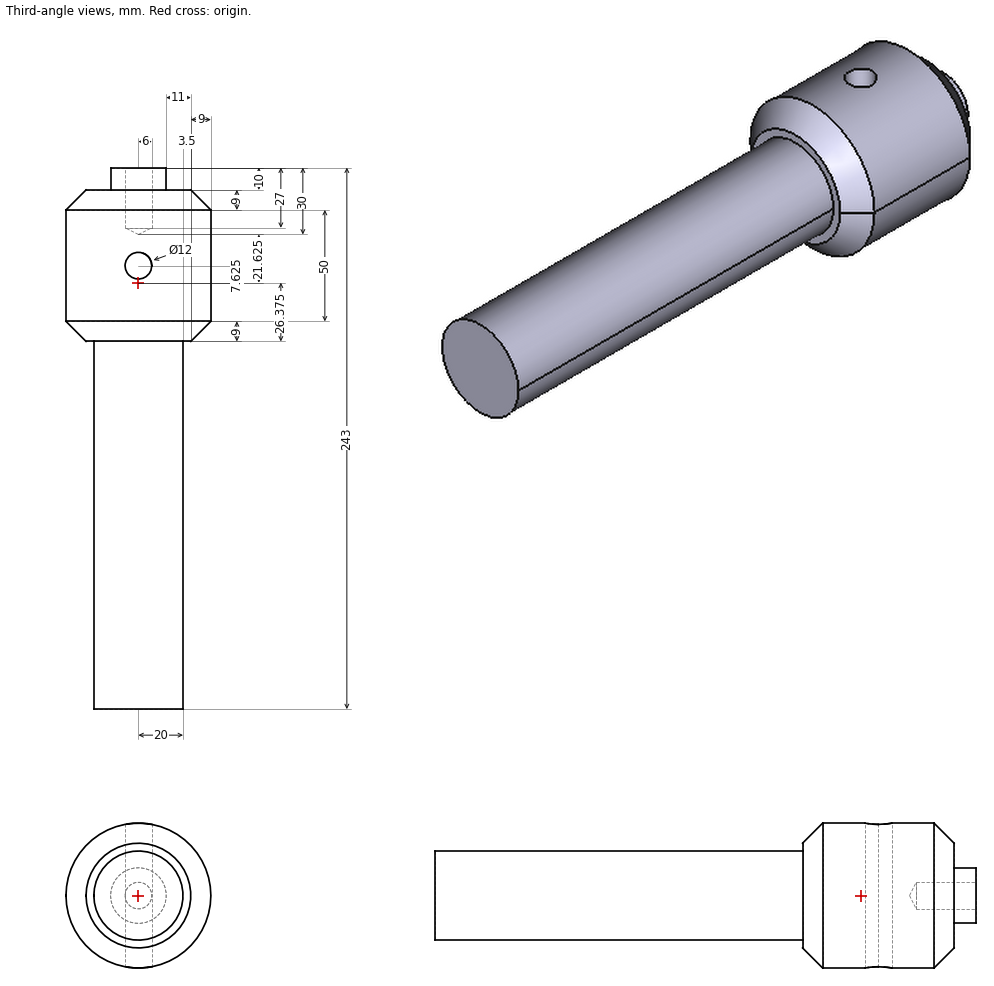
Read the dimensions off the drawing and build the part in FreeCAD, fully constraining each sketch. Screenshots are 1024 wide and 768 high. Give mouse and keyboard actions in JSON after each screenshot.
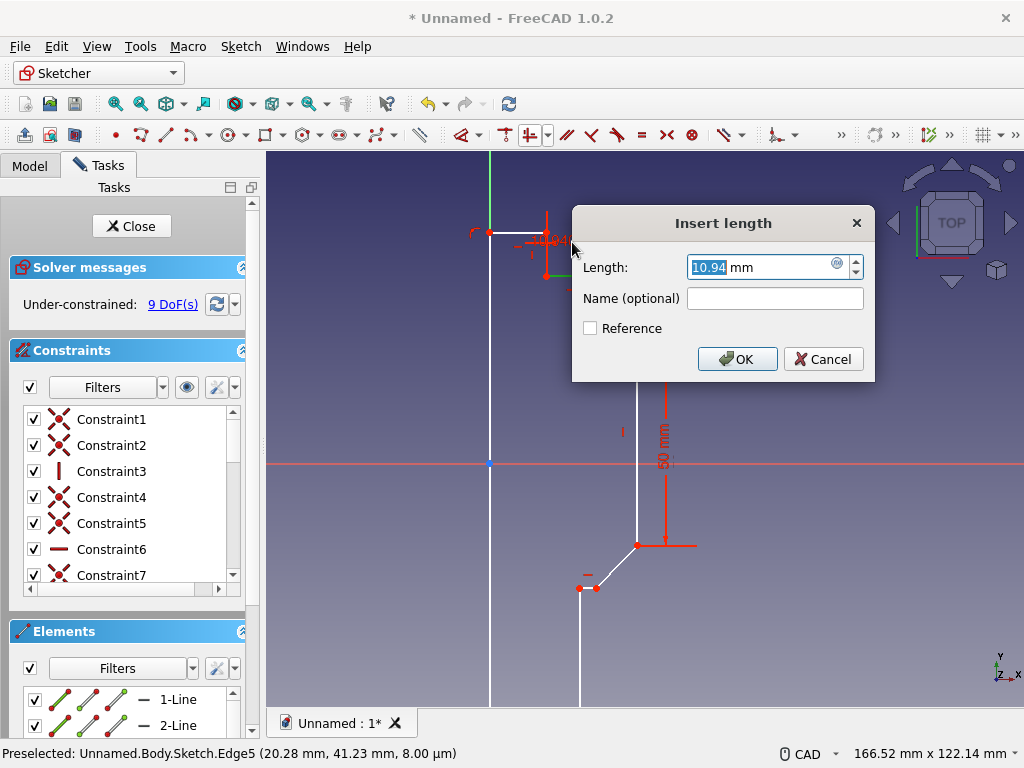
{"action": "type", "text": "11"}
{"action": "key", "text": "Return"}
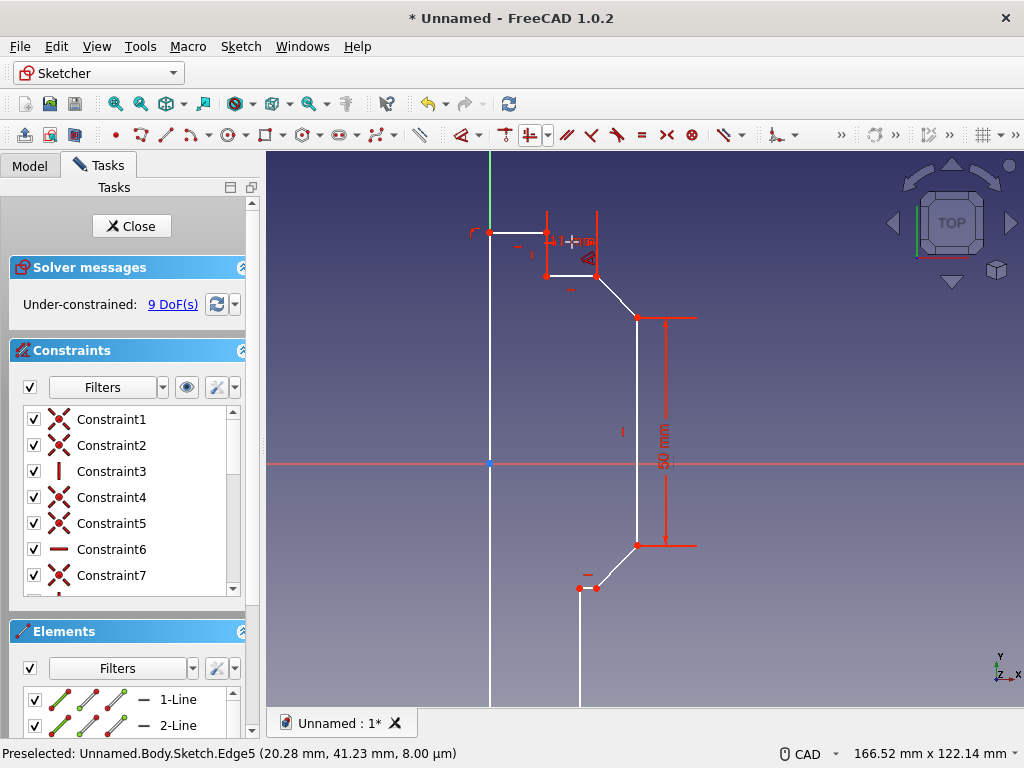
{"action": "left_click", "coordinate": [547, 263]}
{"action": "left_click", "coordinate": [513, 264]}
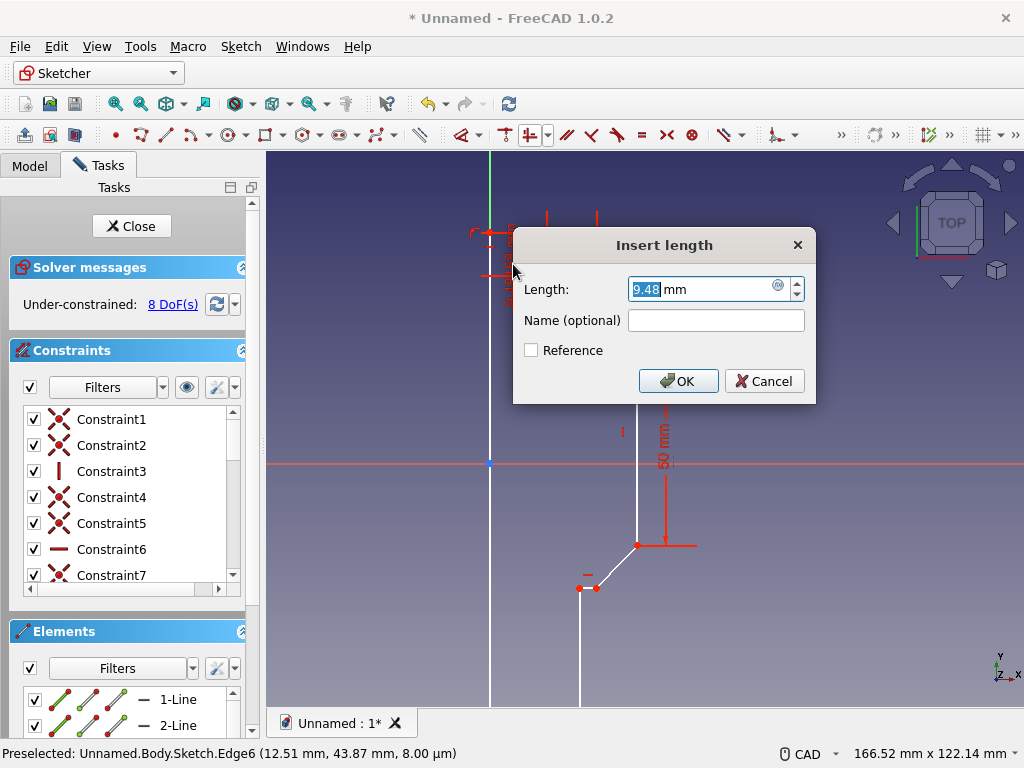
{"action": "type", "text": "10"}
{"action": "key", "text": "Return"}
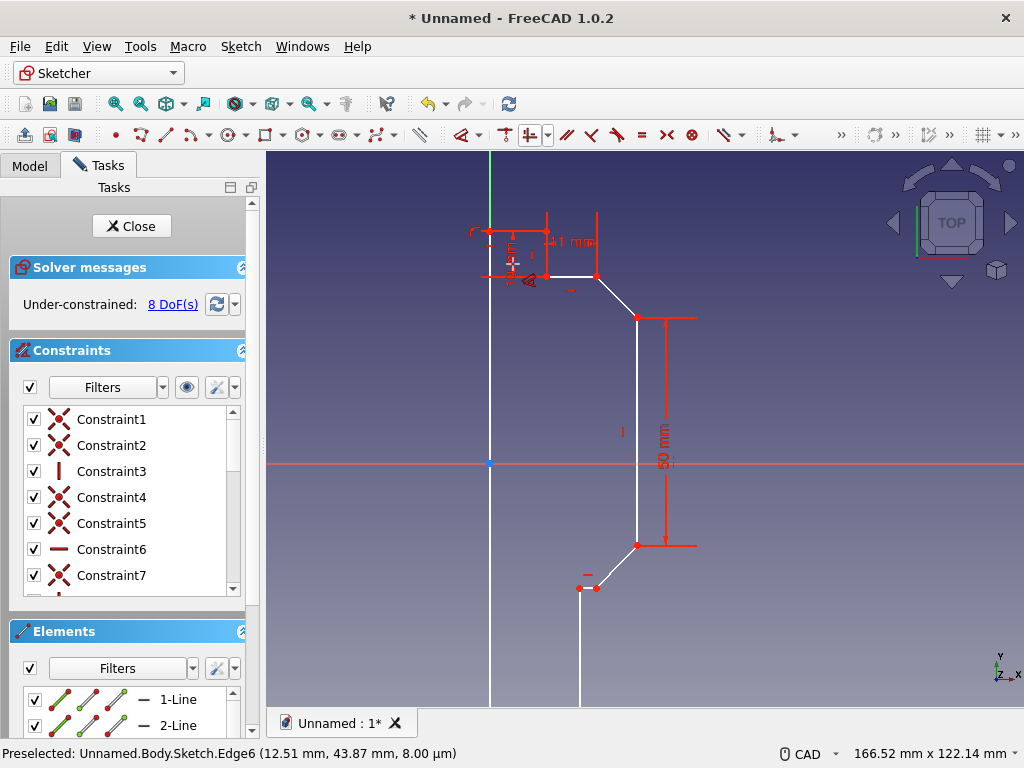
{"action": "scroll", "coordinate": [582, 277], "scroll_direction": "down", "scroll_amount": 6}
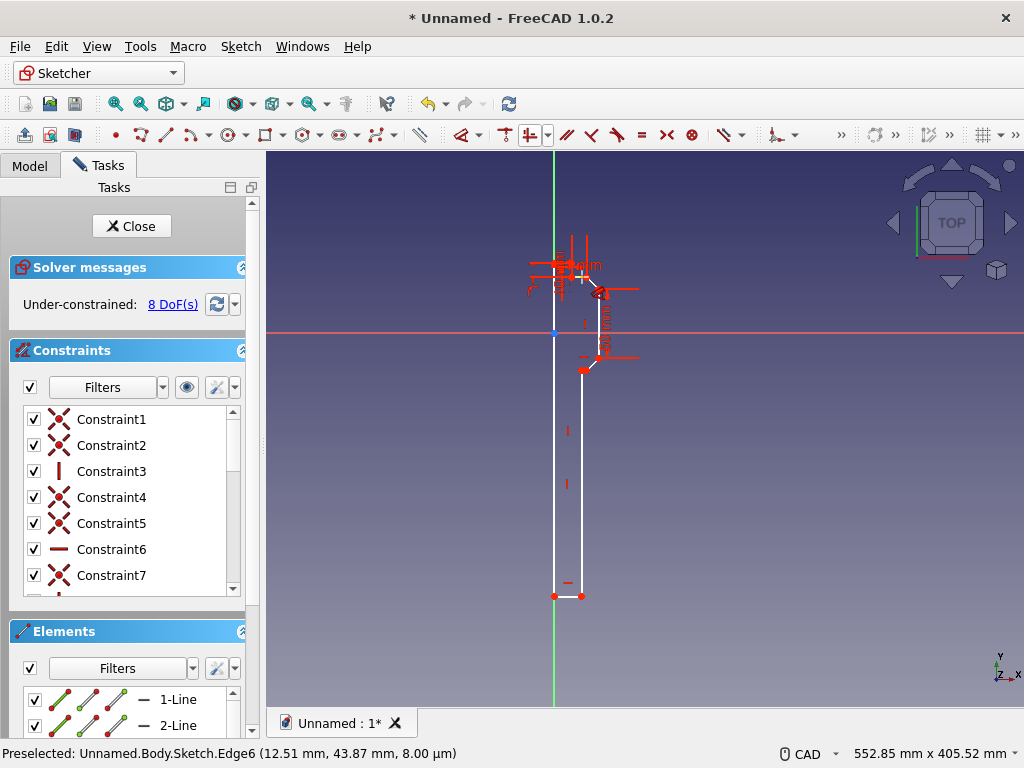
{"action": "scroll", "coordinate": [563, 597], "scroll_direction": "up", "scroll_amount": 3}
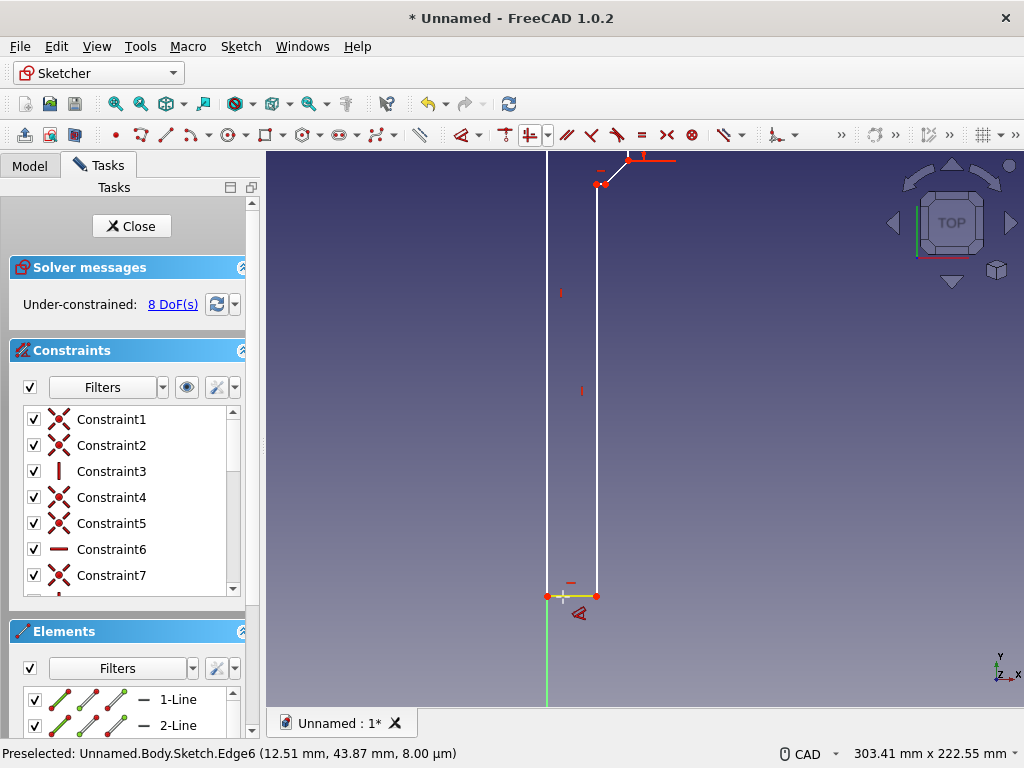
{"action": "left_click", "coordinate": [562, 596]}
{"action": "left_click", "coordinate": [572, 630]}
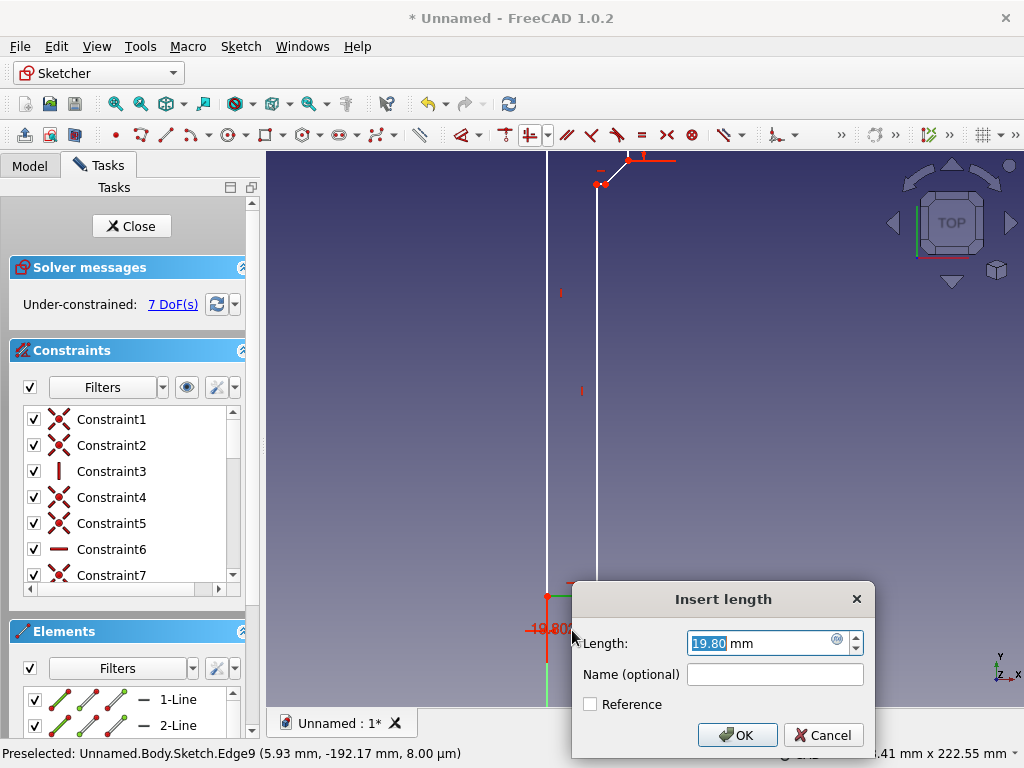
{"action": "type", "text": "20"}
{"action": "key", "text": "Return"}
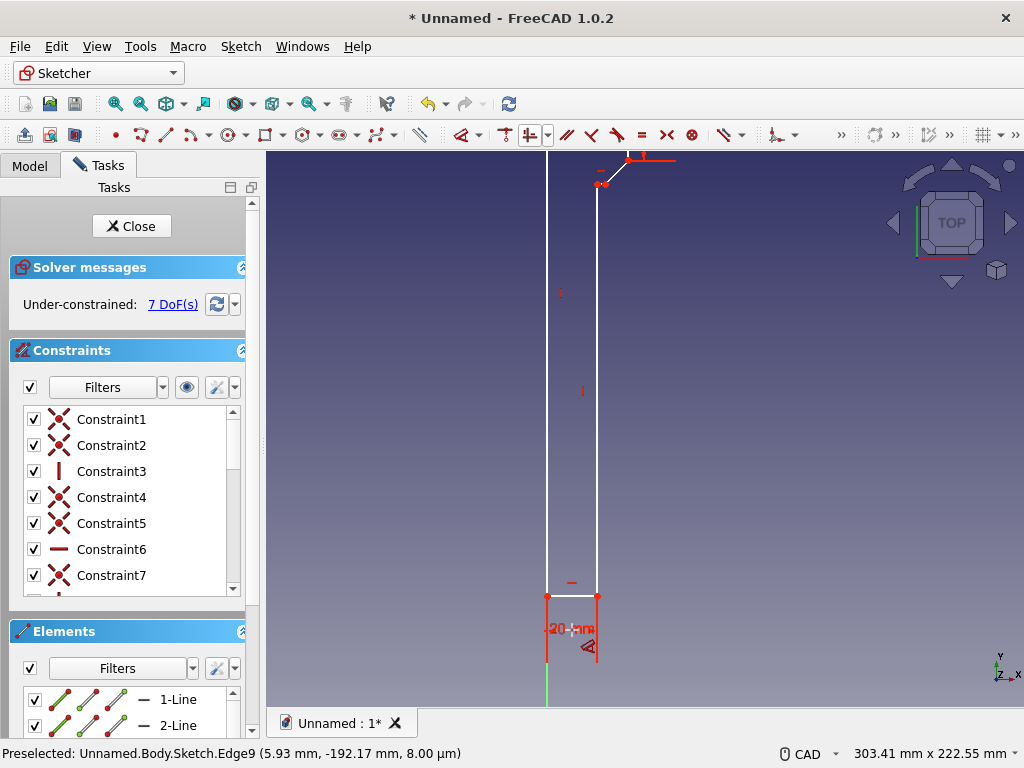
{"action": "scroll", "coordinate": [563, 597], "scroll_direction": "down", "scroll_amount": 3}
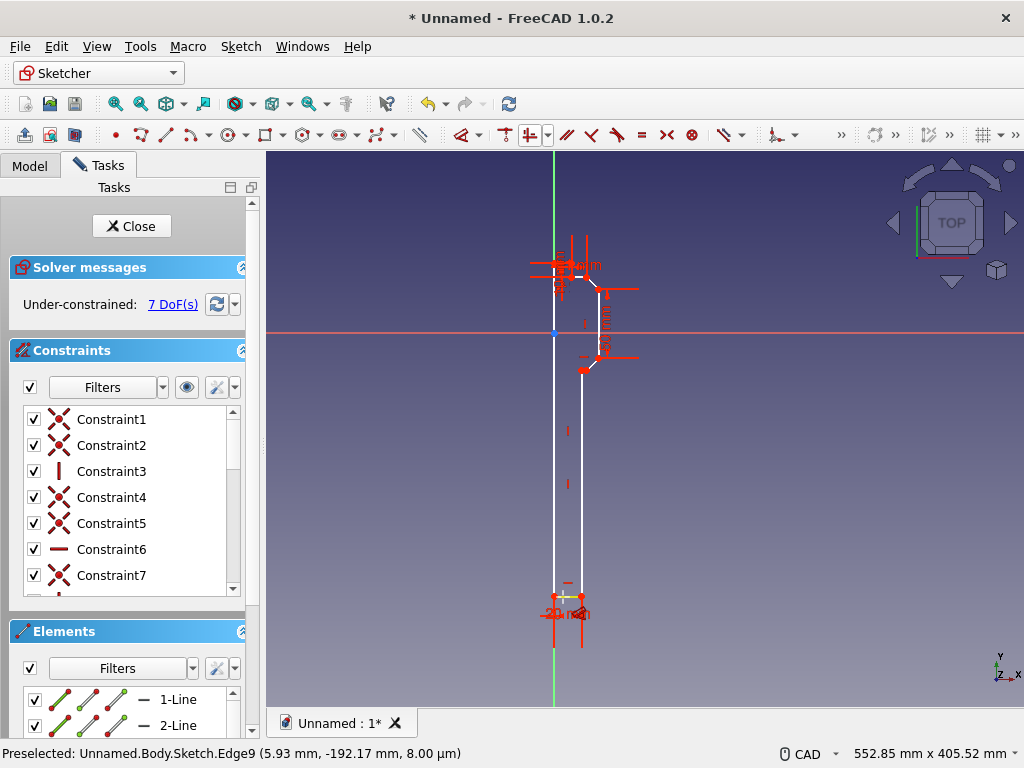
{"action": "scroll", "coordinate": [590, 367], "scroll_direction": "up", "scroll_amount": 6}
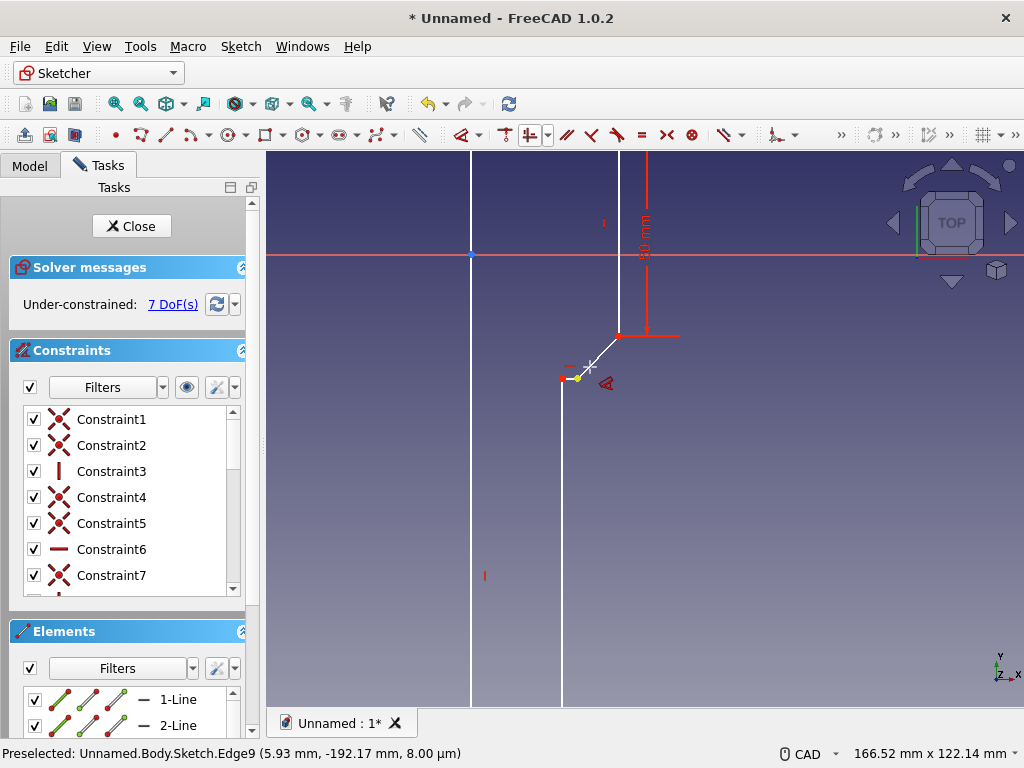
{"action": "left_click", "coordinate": [590, 366]}
{"action": "left_click", "coordinate": [598, 302]}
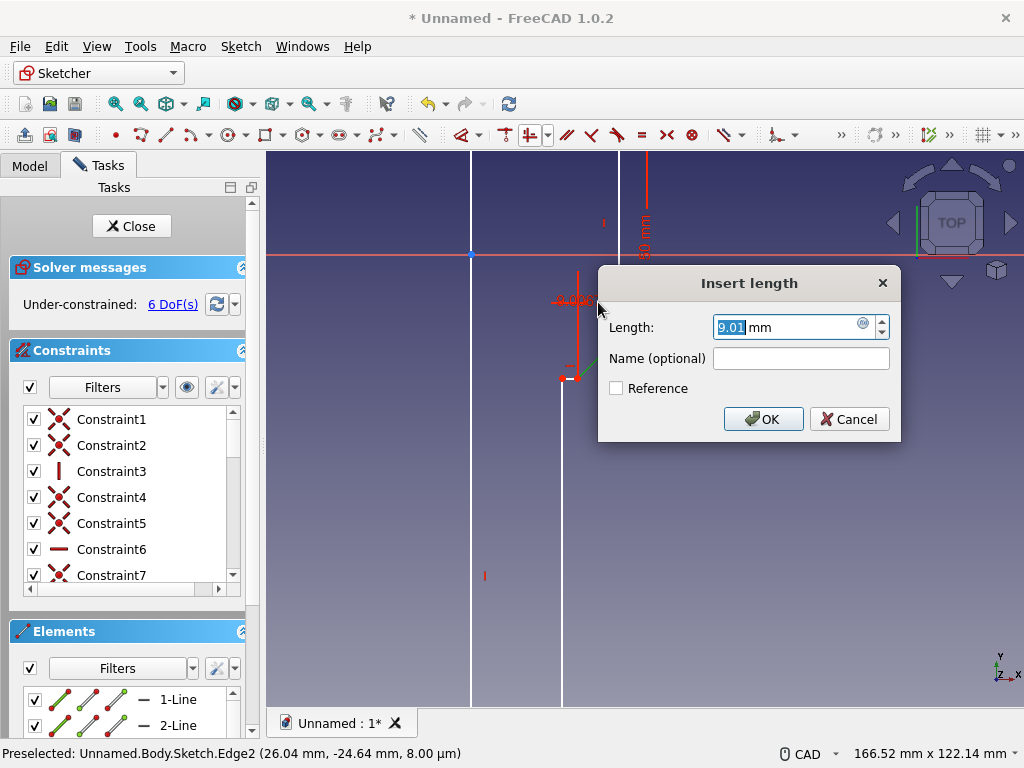
{"action": "type", "text": "9"}
{"action": "key", "text": "Return"}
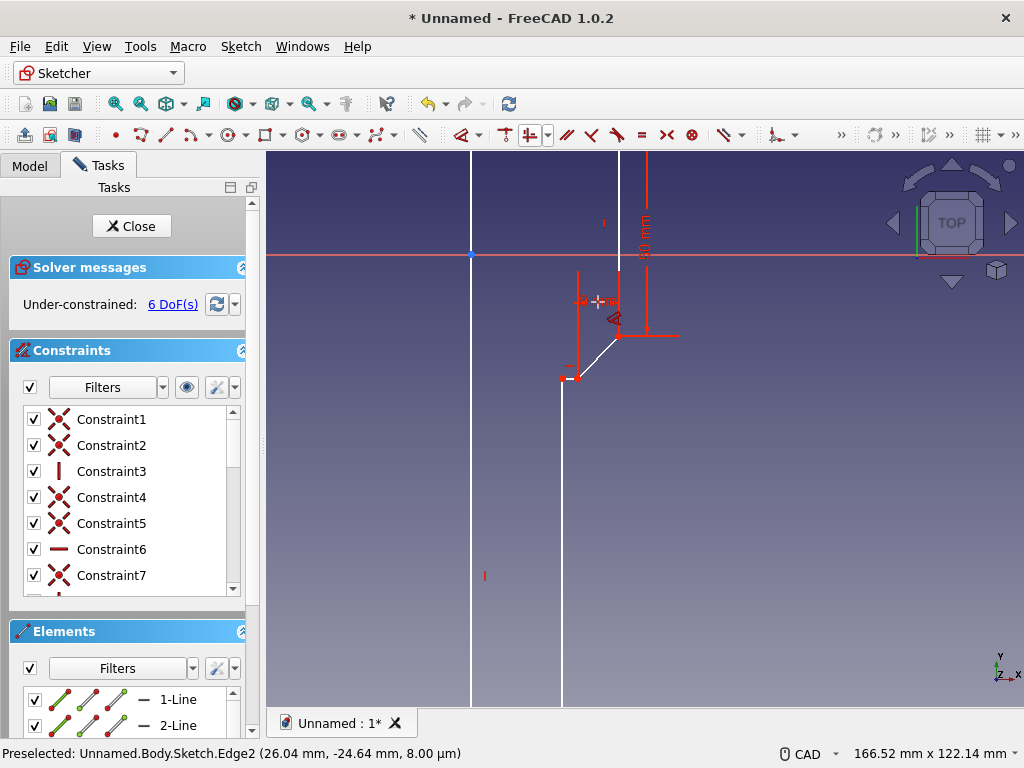
{"action": "left_click", "coordinate": [590, 366]}
{"action": "left_click", "coordinate": [653, 358]}